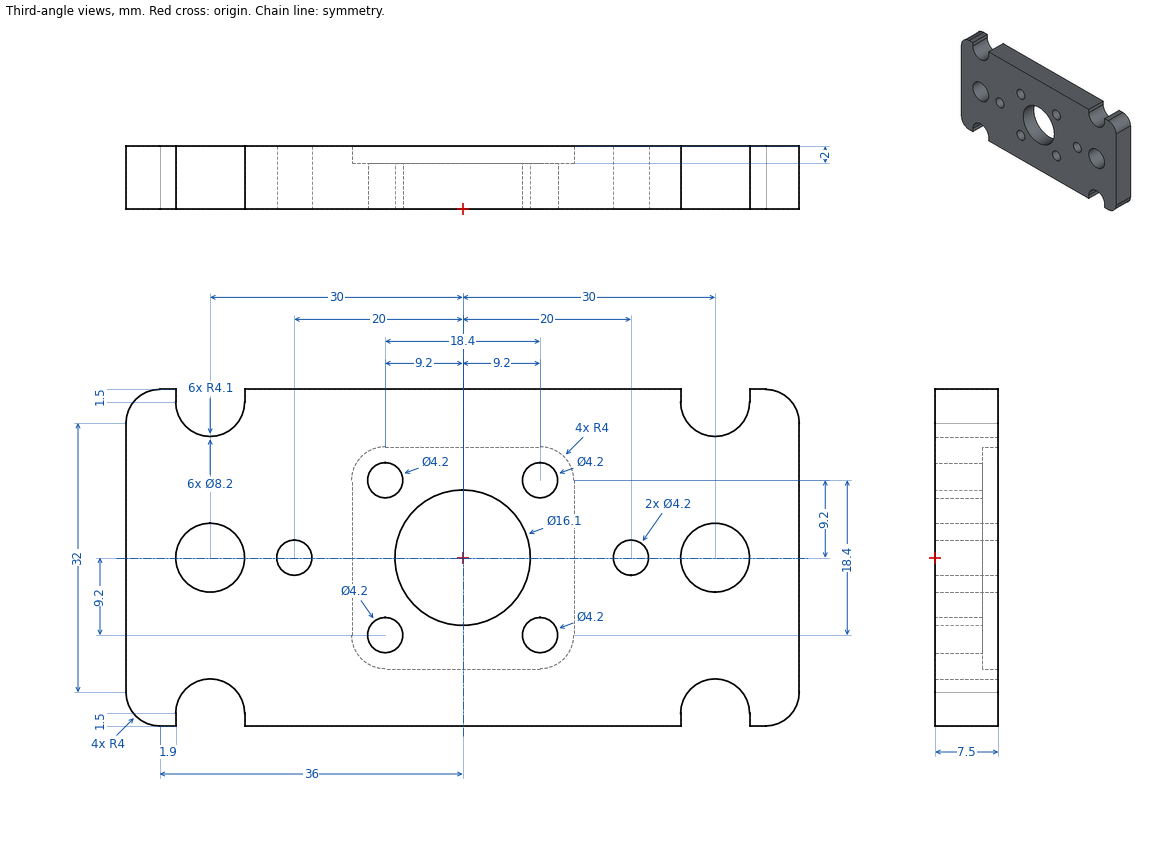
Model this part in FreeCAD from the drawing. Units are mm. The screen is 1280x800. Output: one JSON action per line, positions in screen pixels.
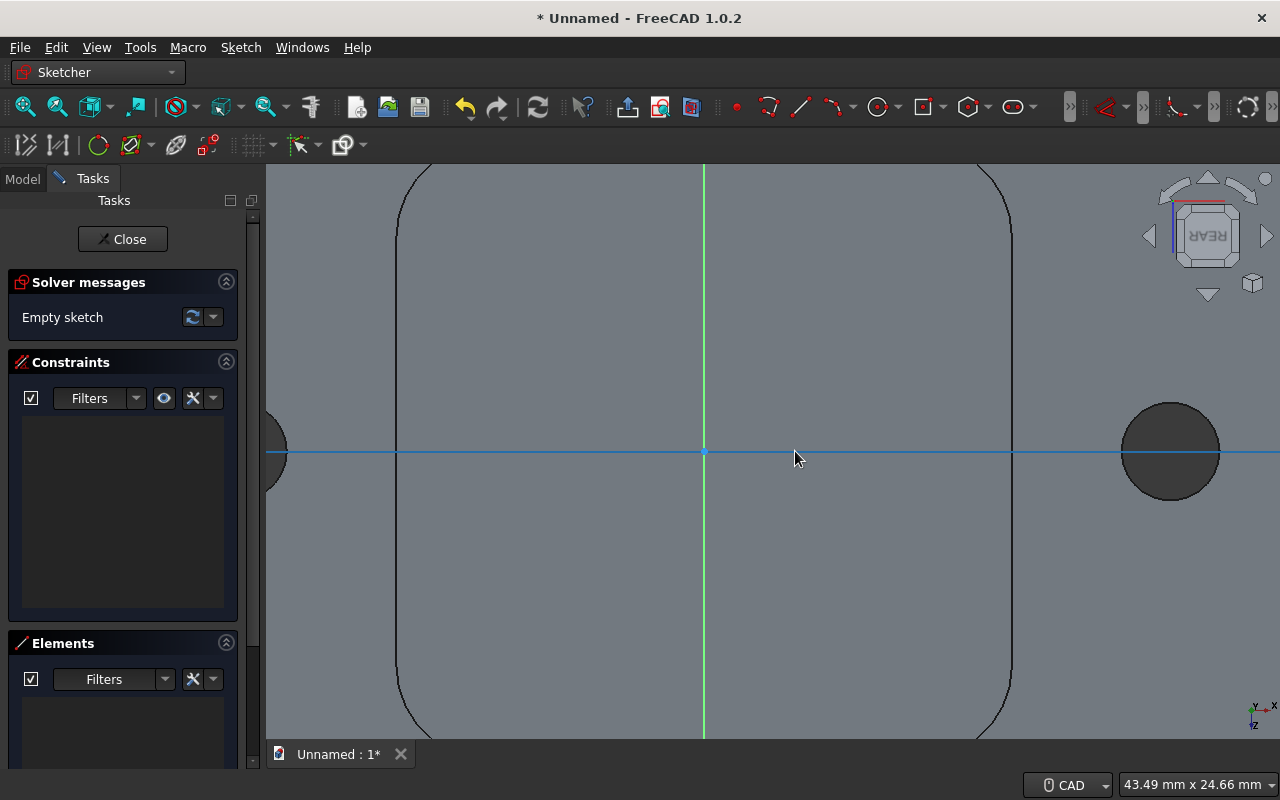
{"action": "left_click", "coordinate": [878, 108]}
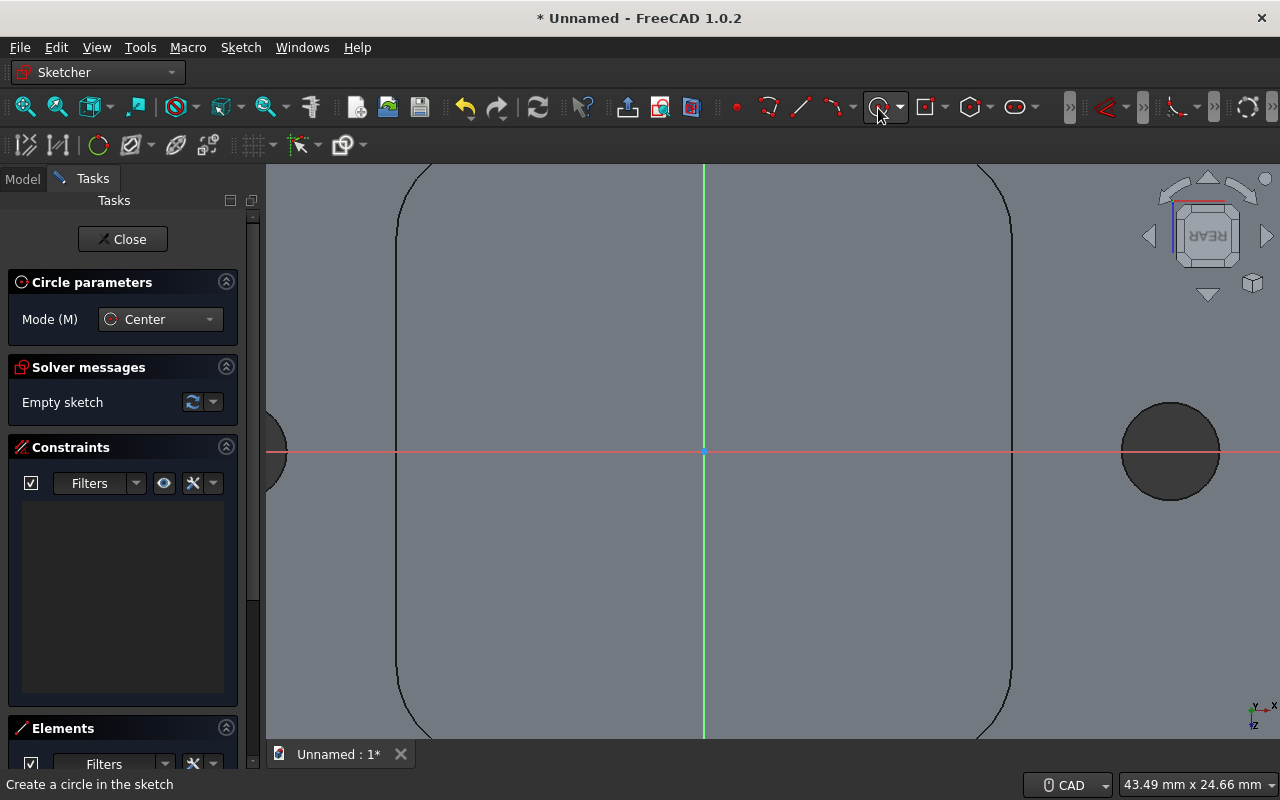
{"action": "left_click", "coordinate": [704, 451]}
{"action": "mouse_move", "coordinate": [837, 319]}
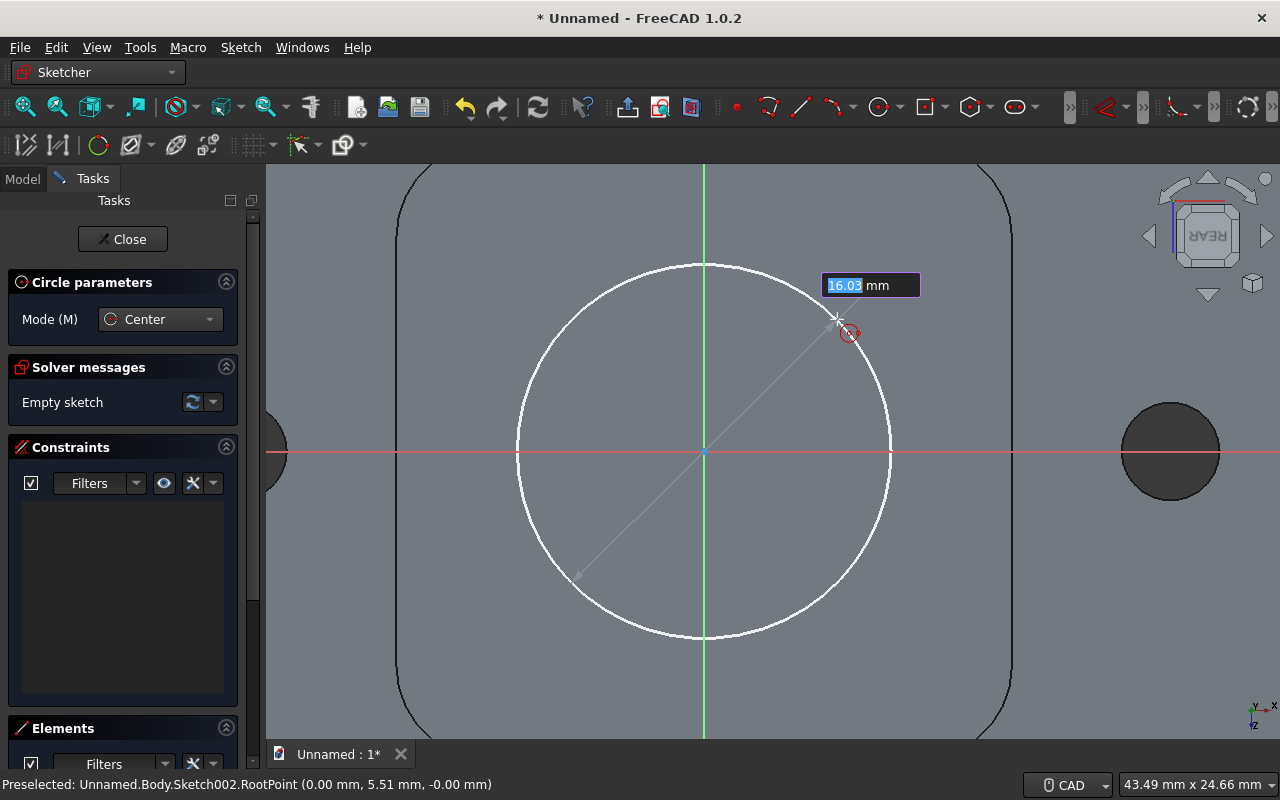
{"action": "type", "text": "16.1"}
{"action": "key", "text": "Return"}
{"action": "key", "text": "Escape"}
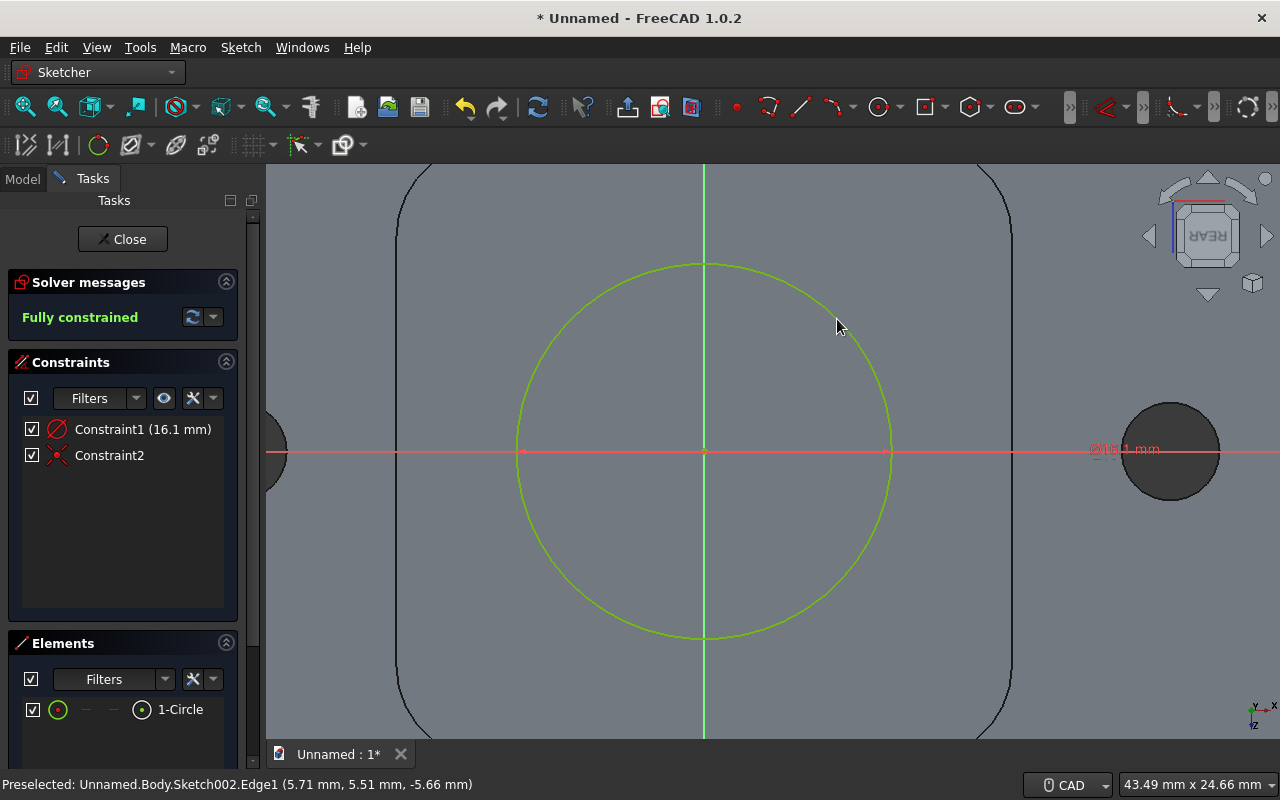
{"action": "left_click", "coordinate": [123, 239]}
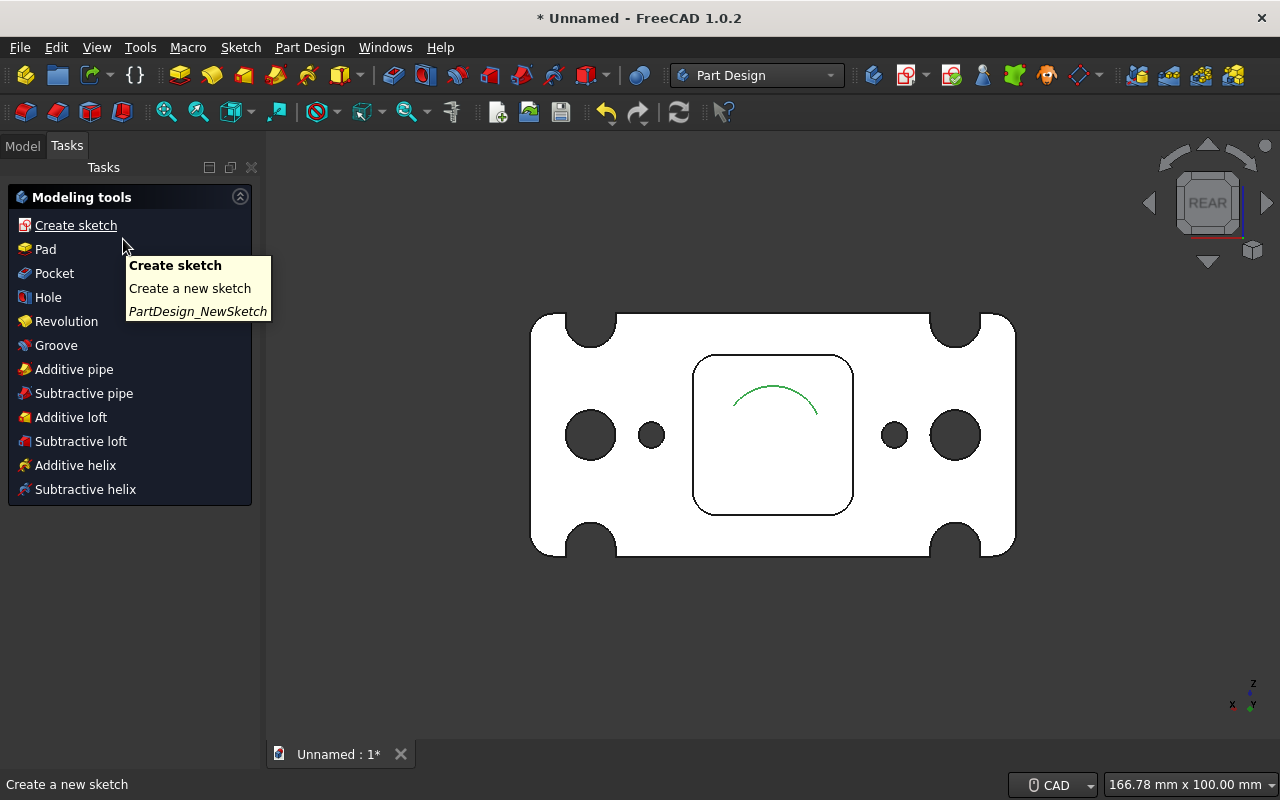
{"action": "left_click", "coordinate": [394, 76]}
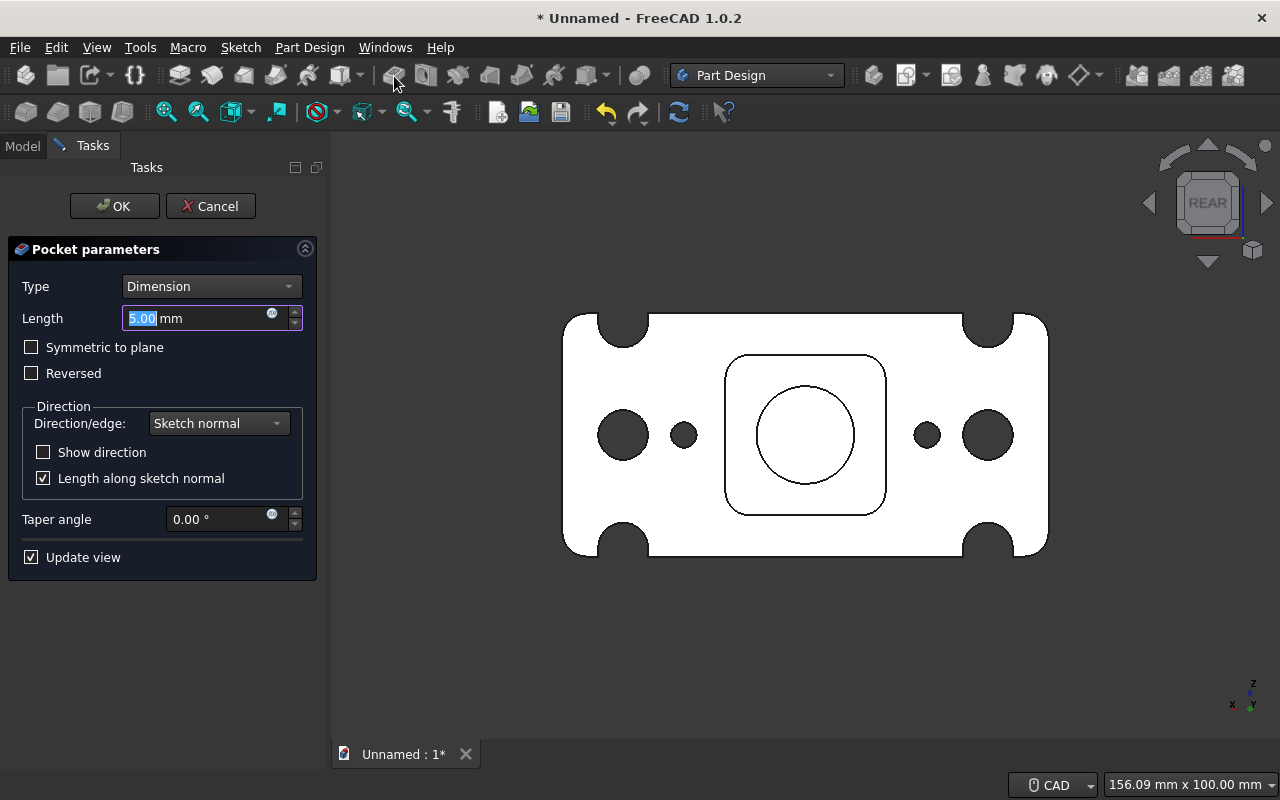
{"action": "left_click", "coordinate": [212, 286]}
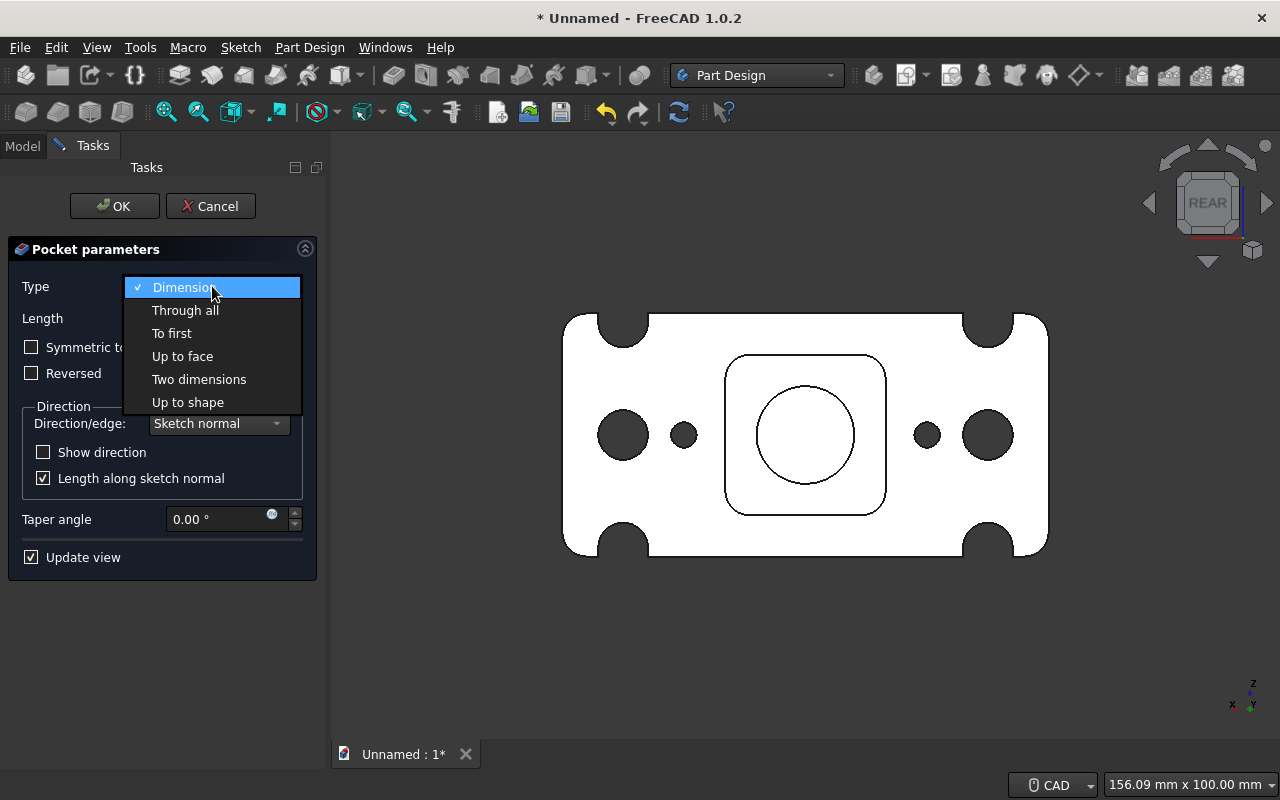
{"action": "left_click", "coordinate": [212, 334]}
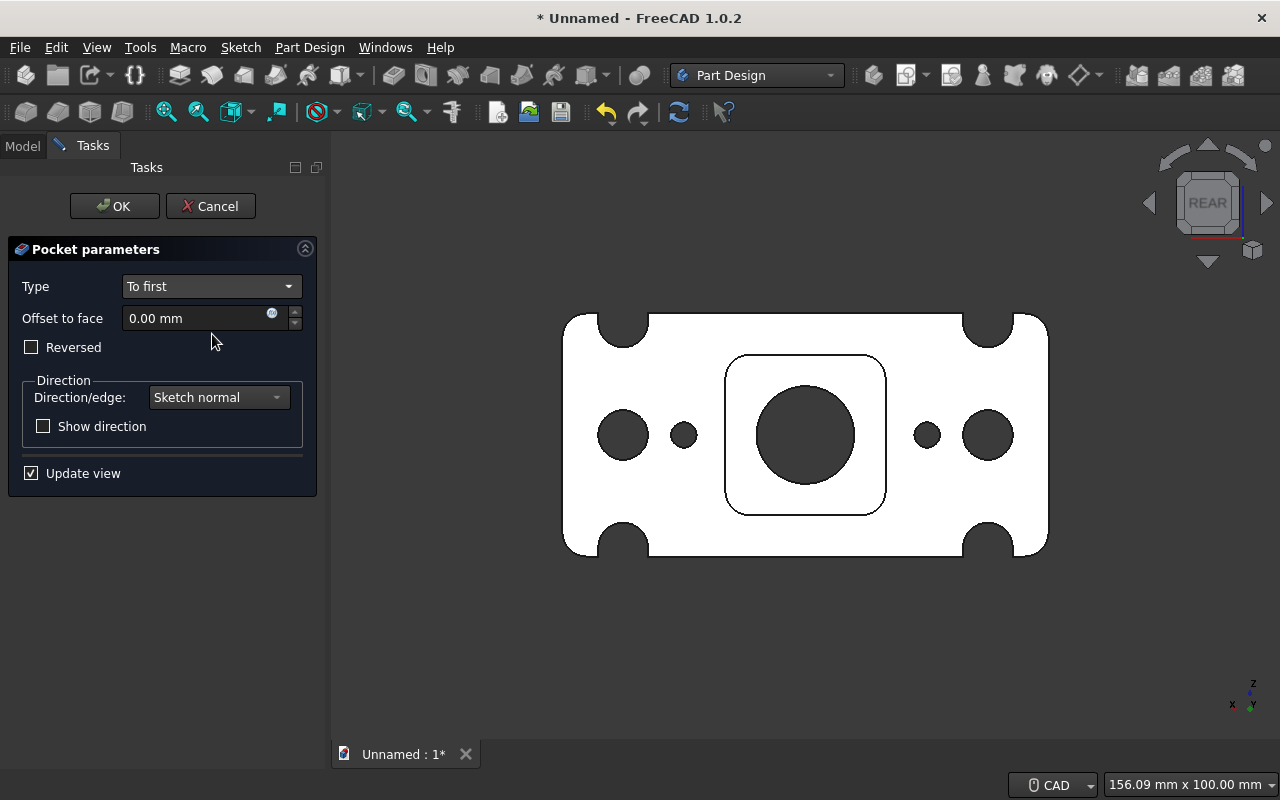
{"action": "left_click", "coordinate": [115, 206]}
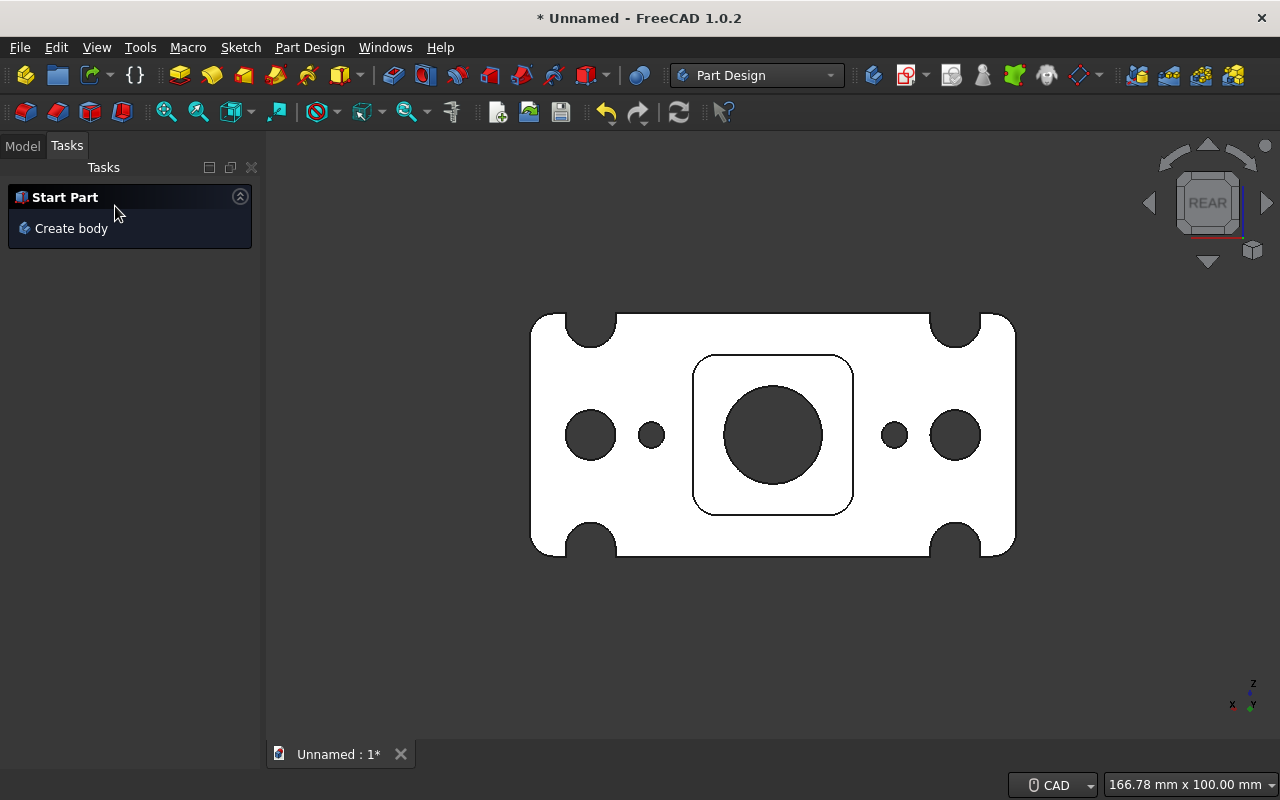
{"action": "left_click", "coordinate": [819, 388]}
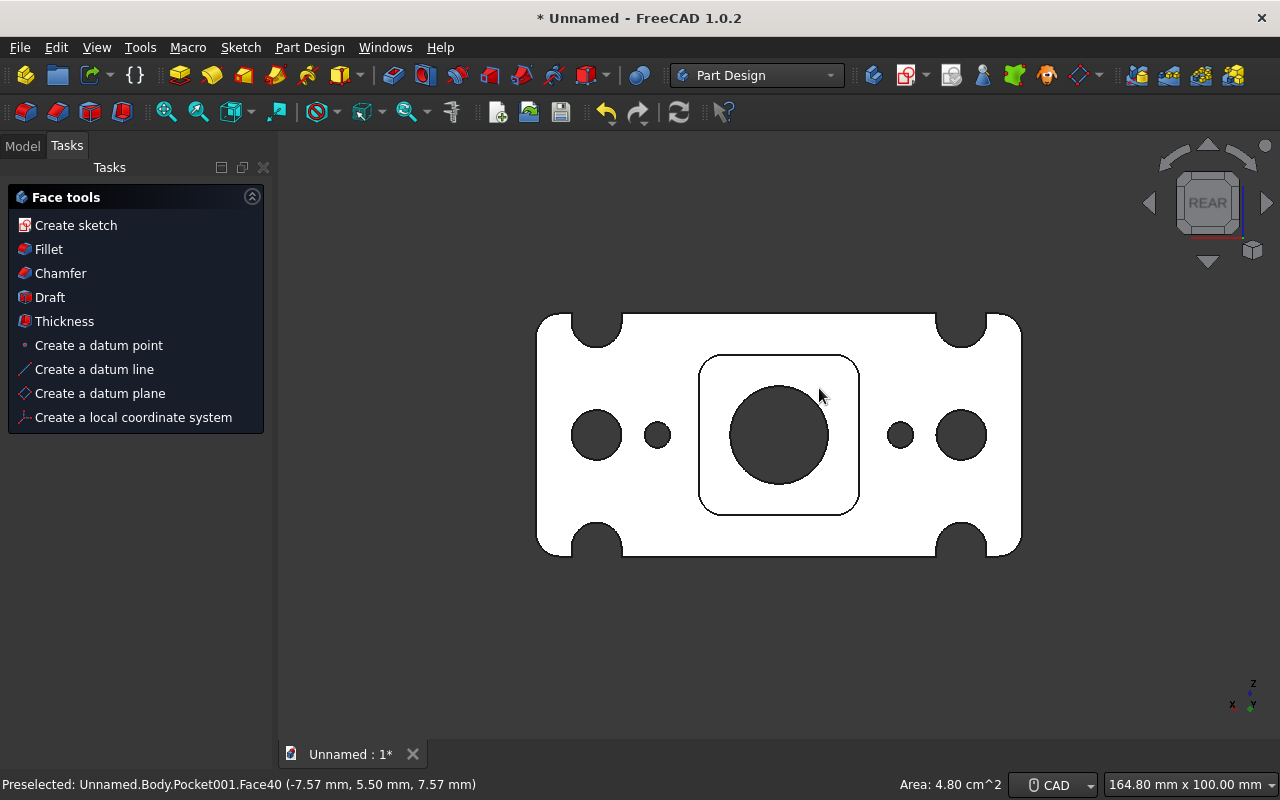
{"action": "left_click", "coordinate": [906, 76]}